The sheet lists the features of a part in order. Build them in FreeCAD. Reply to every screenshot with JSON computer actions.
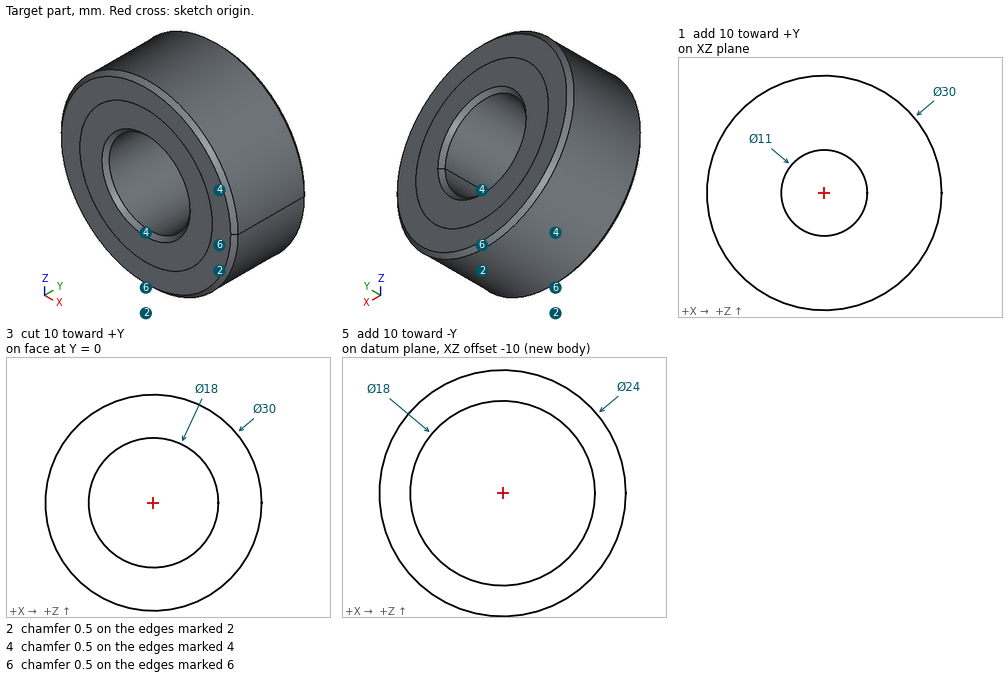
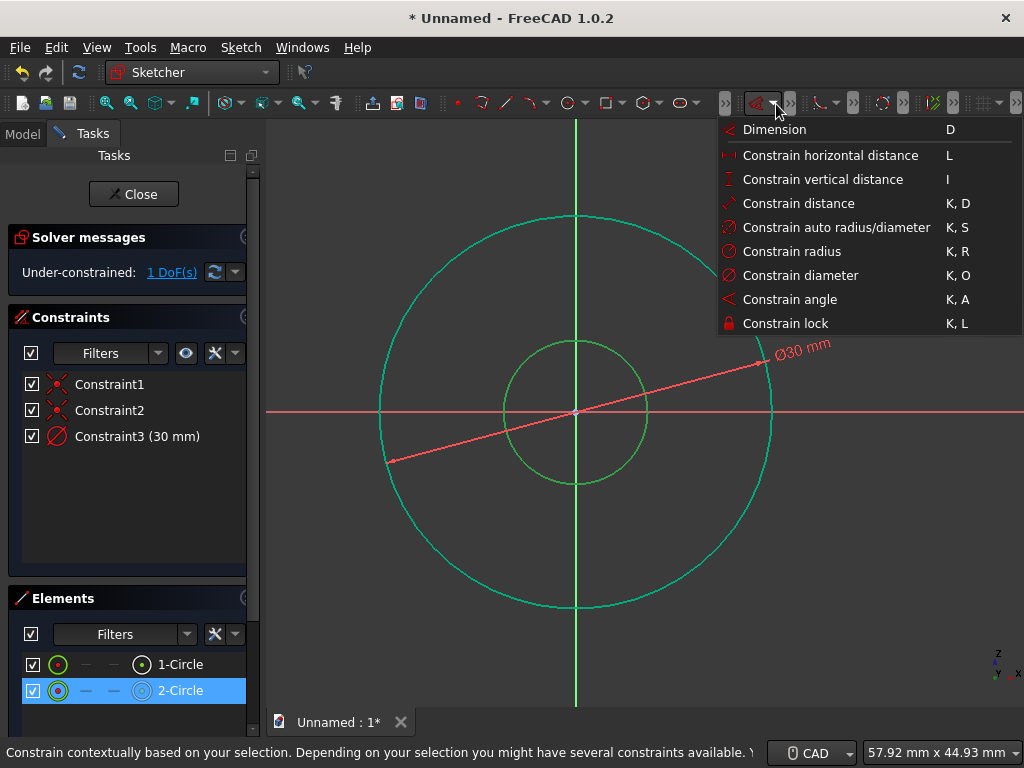
{"action": "left_click", "coordinate": [870, 275]}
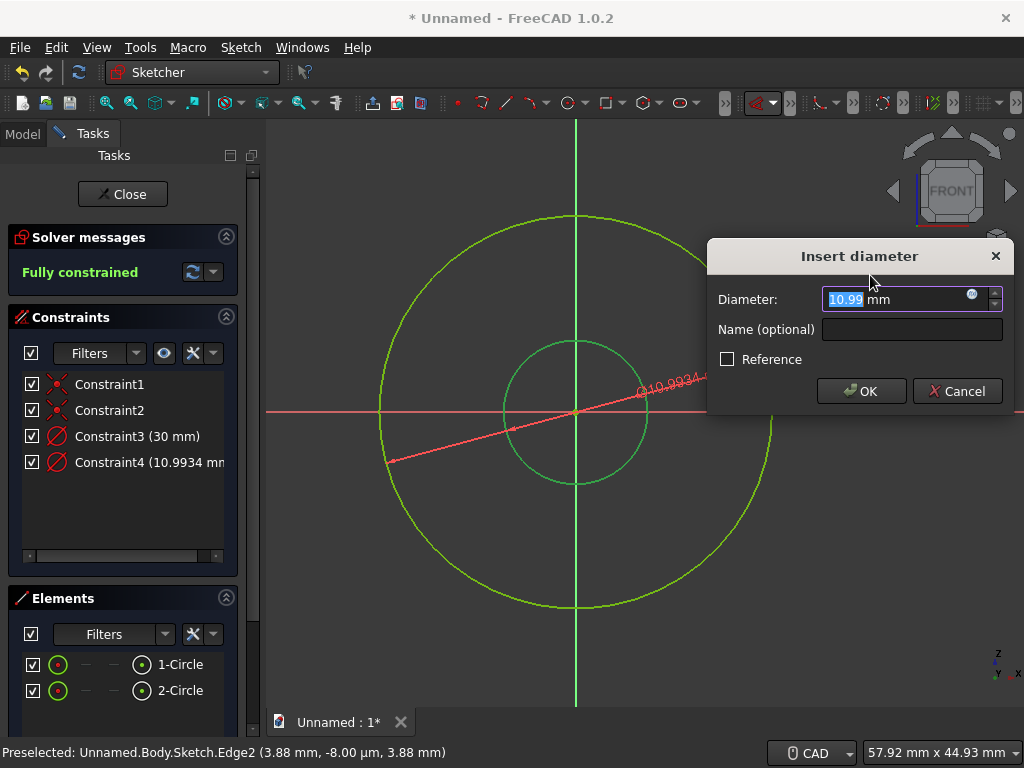
{"action": "type", "text": "11"}
{"action": "key", "text": "Return"}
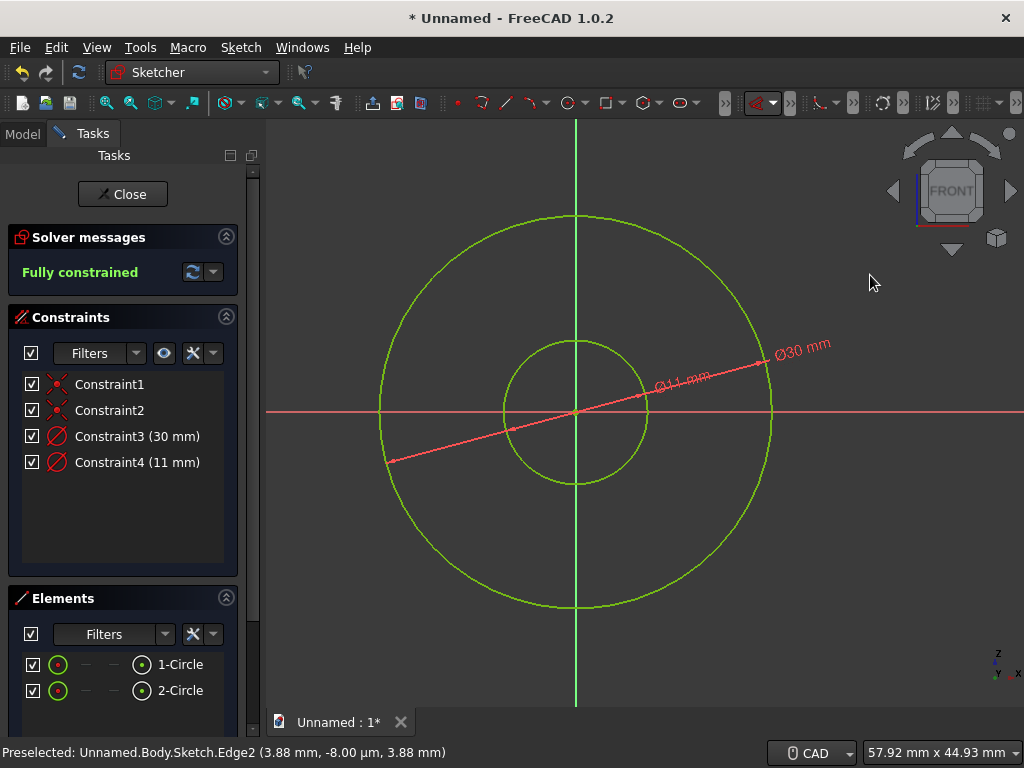
{"action": "left_click", "coordinate": [123, 194]}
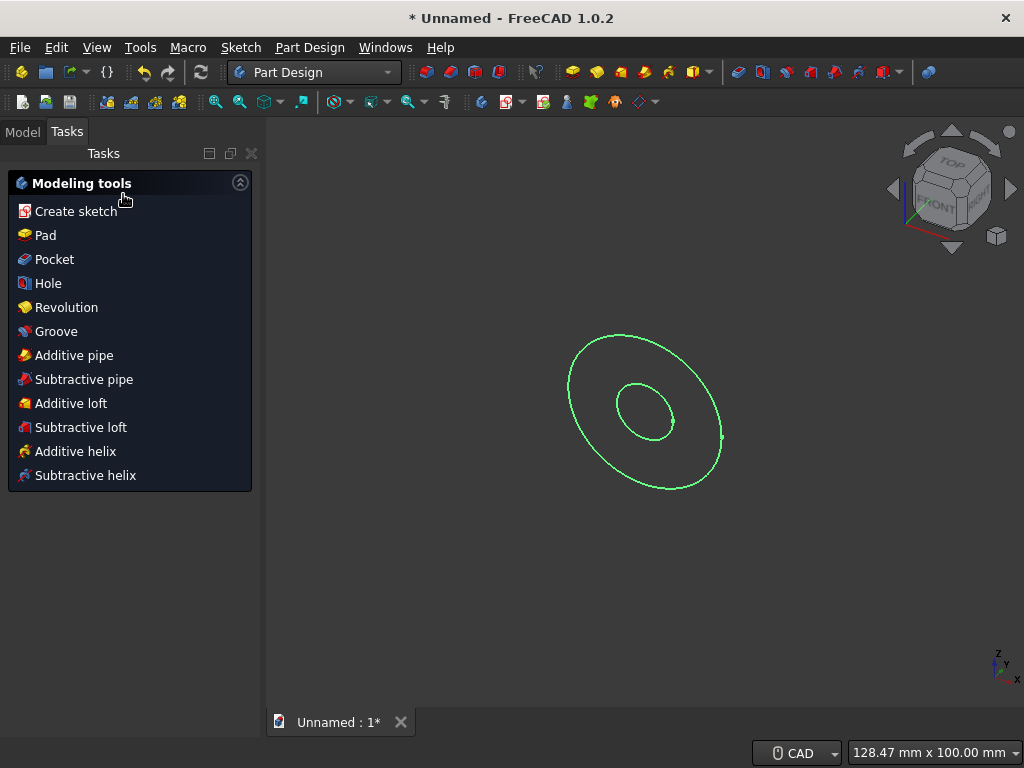
{"action": "left_click", "coordinate": [574, 72]}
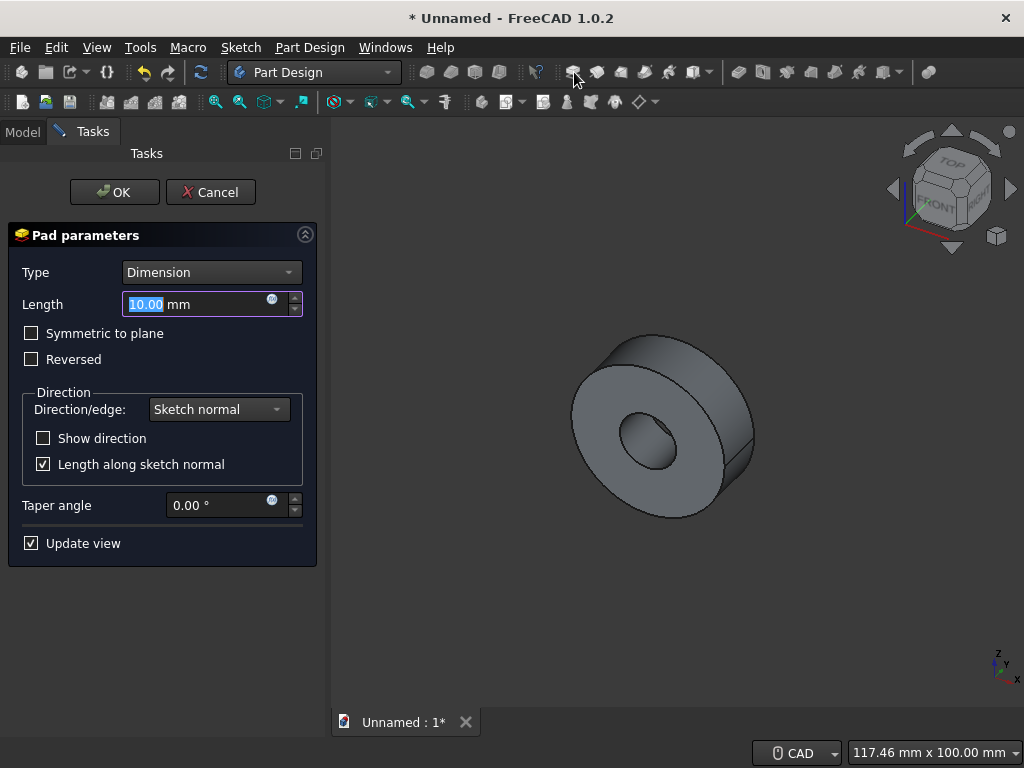
{"action": "type", "text": "10"}
{"action": "key", "text": "Tab"}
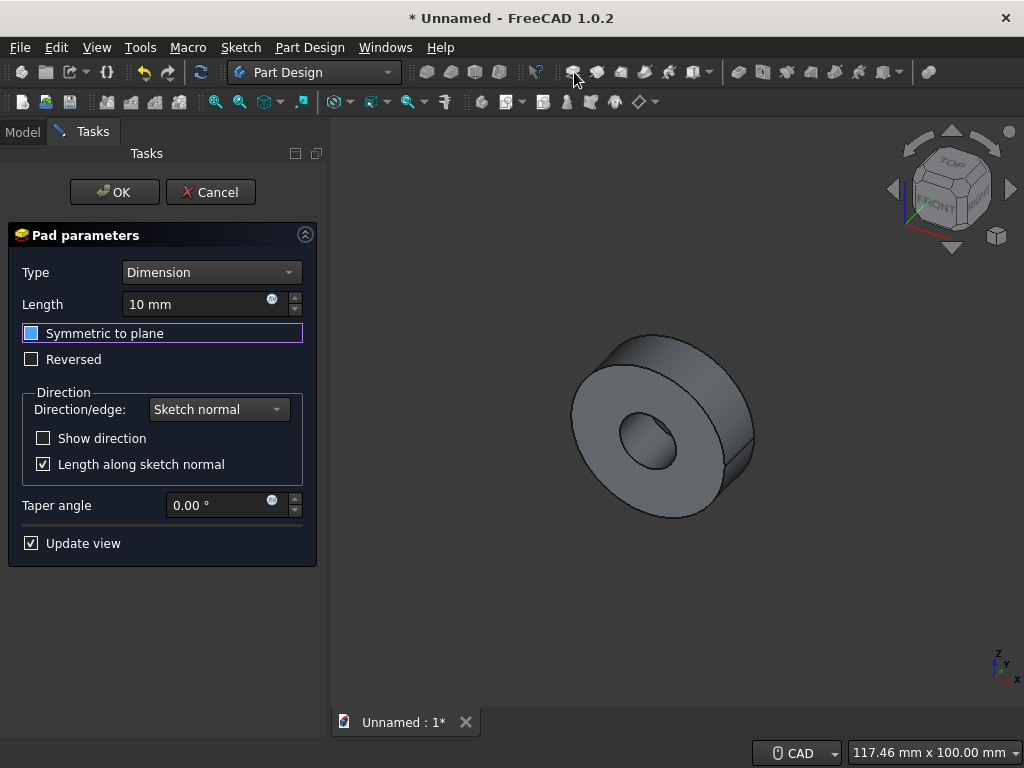
{"action": "left_click", "coordinate": [30, 359]}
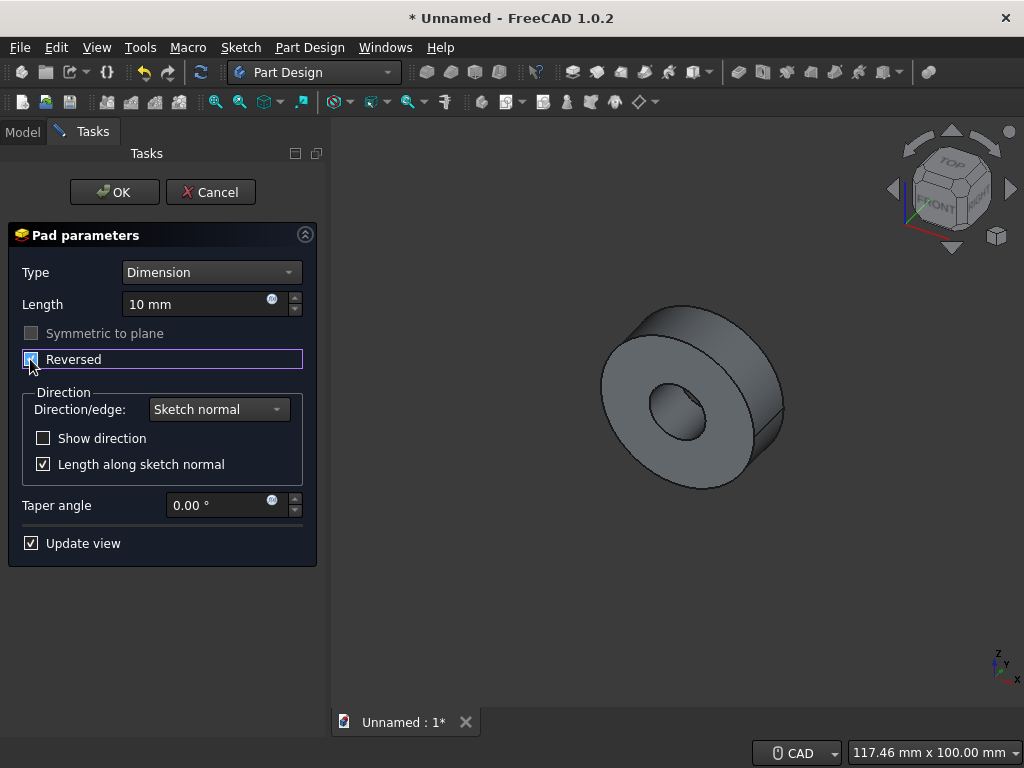
{"action": "left_click", "coordinate": [115, 192]}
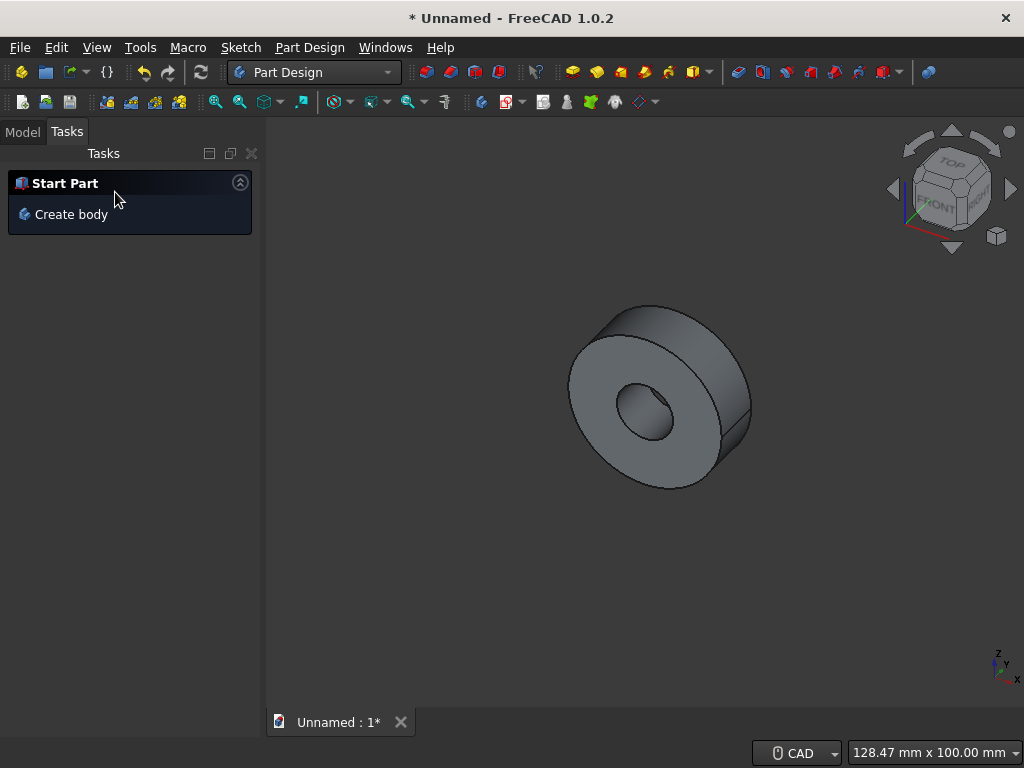
{"action": "left_click", "coordinate": [216, 102]}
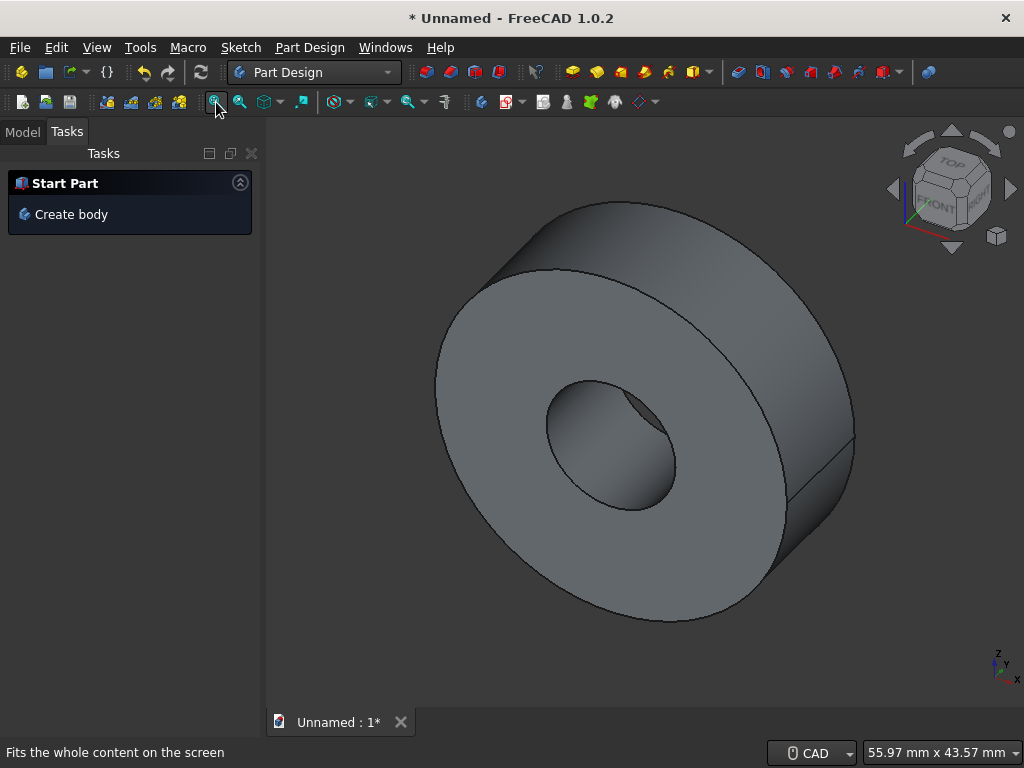
{"action": "left_click", "coordinate": [469, 300]}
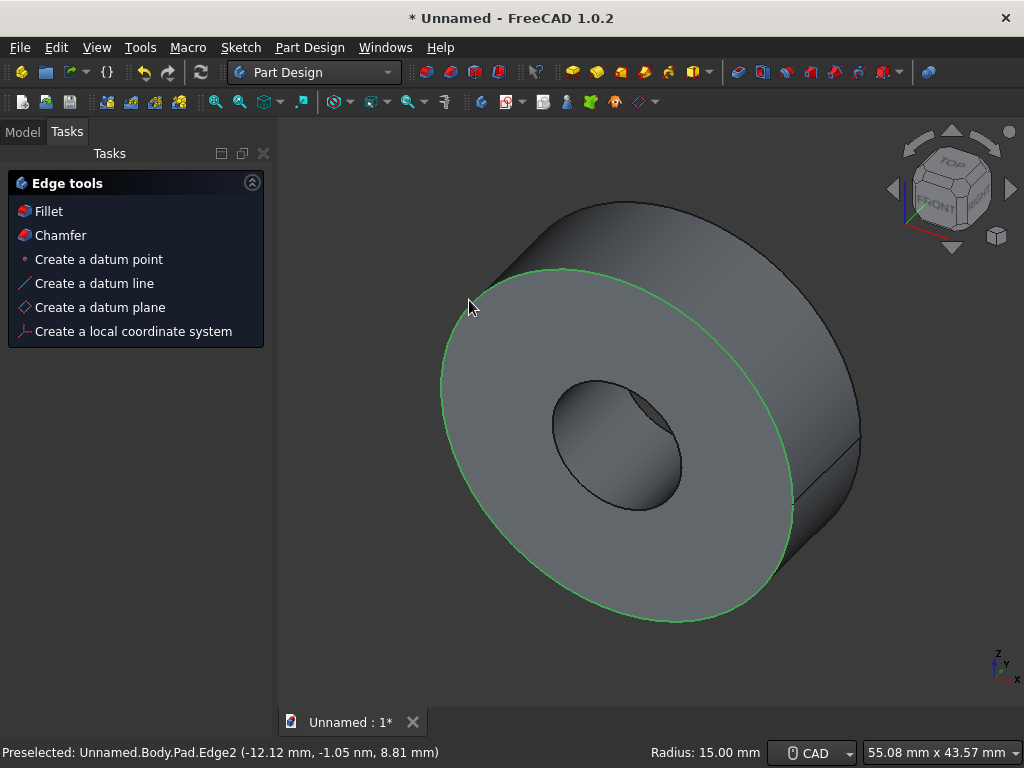
{"action": "key", "text": "0"}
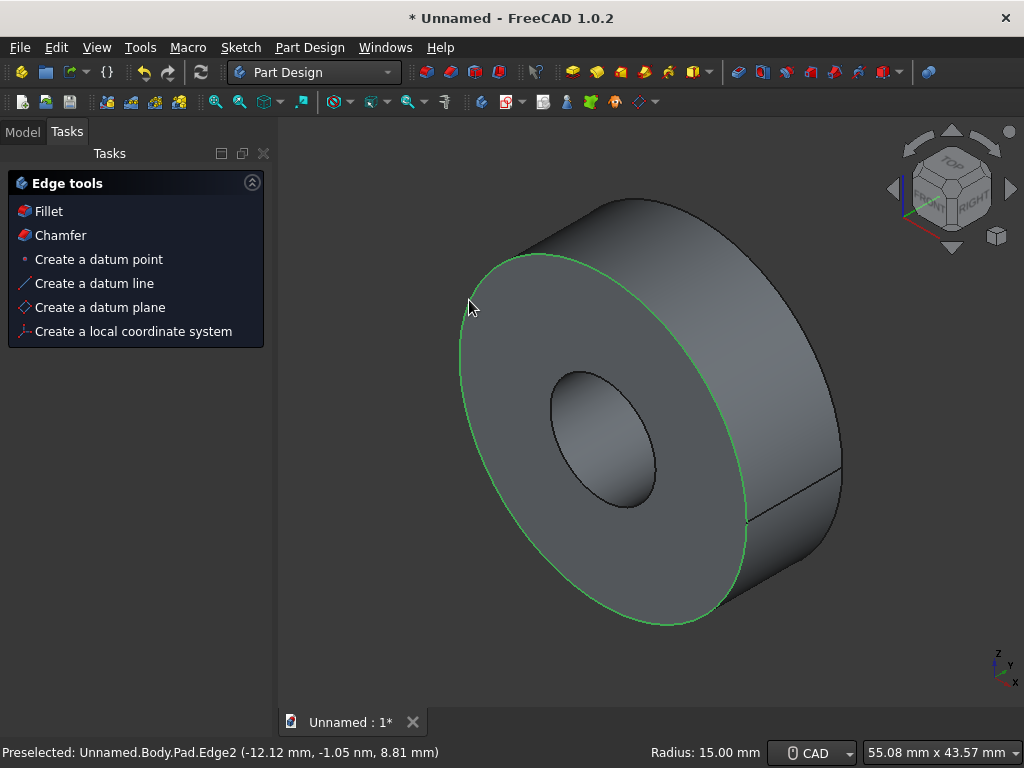
{"action": "key", "text": "2"}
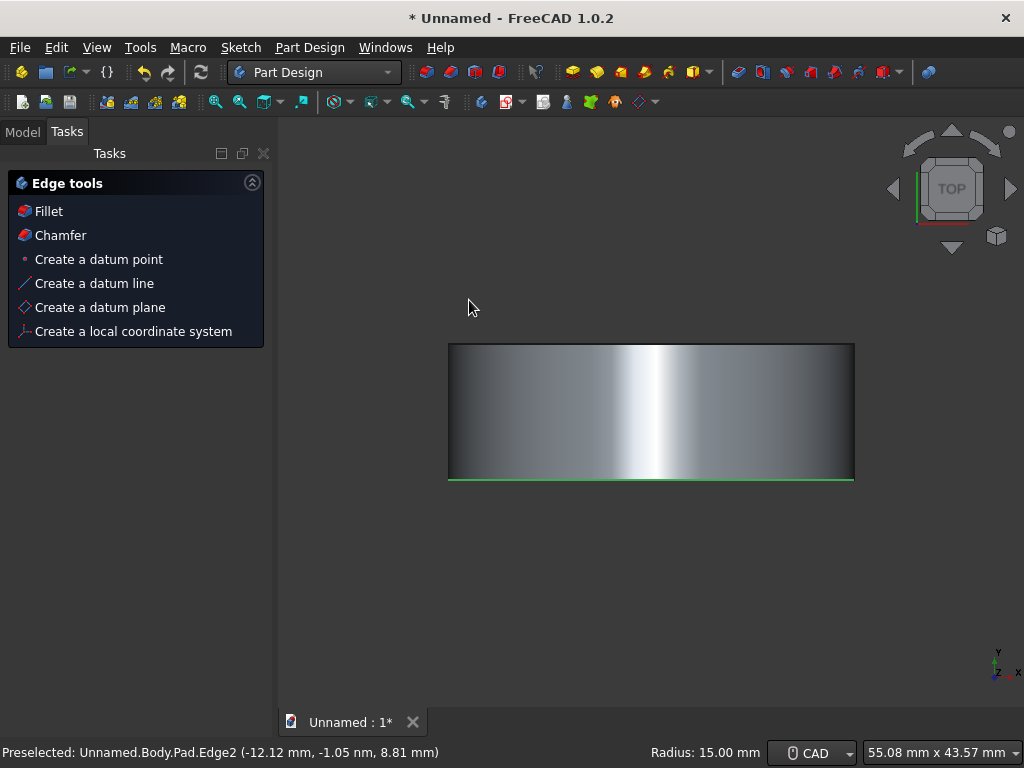
{"action": "left_click", "coordinate": [487, 343], "text": "ctrl"}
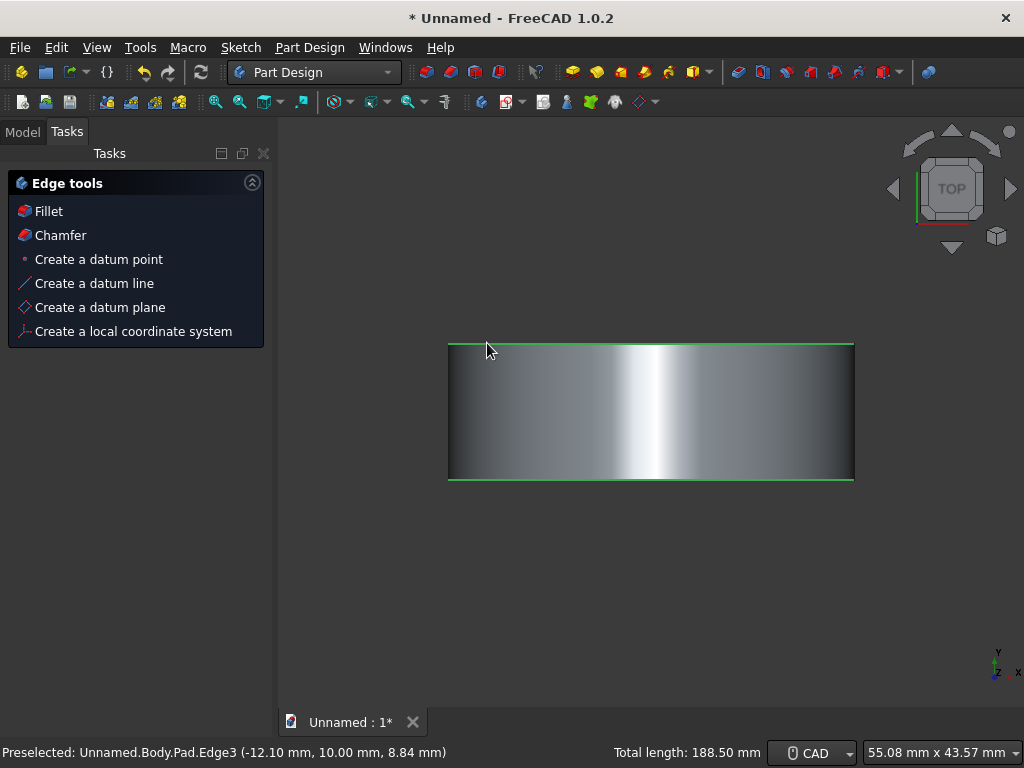
{"action": "left_click", "coordinate": [452, 72]}